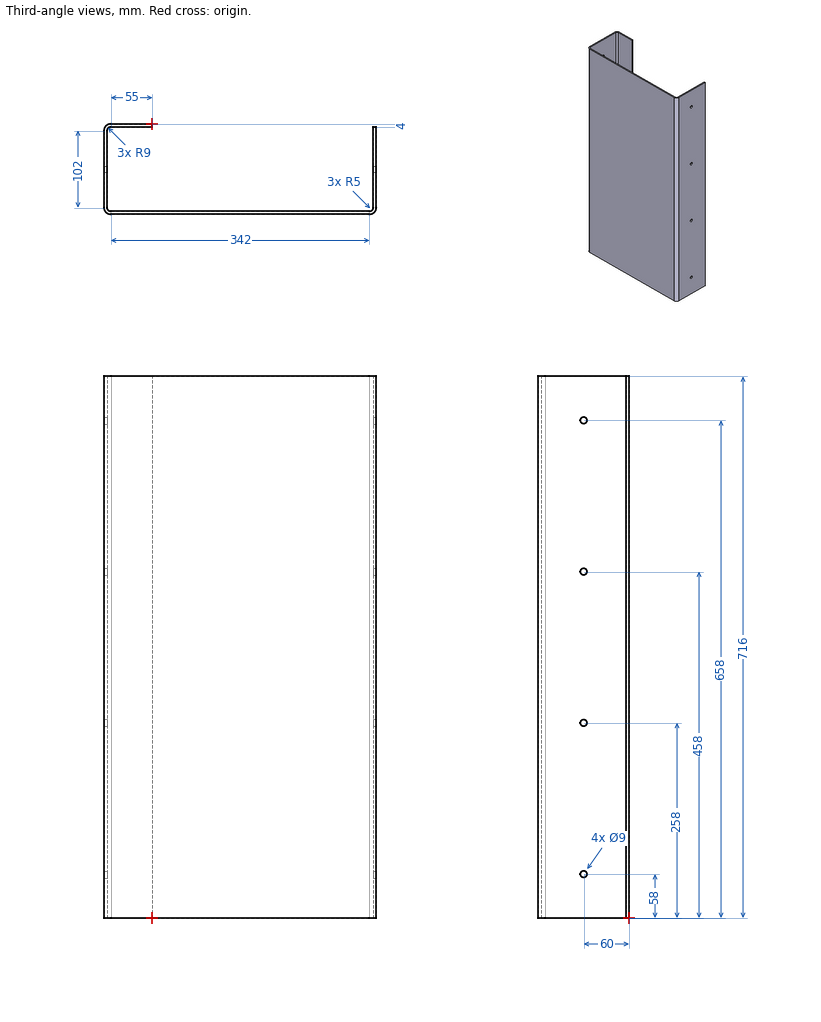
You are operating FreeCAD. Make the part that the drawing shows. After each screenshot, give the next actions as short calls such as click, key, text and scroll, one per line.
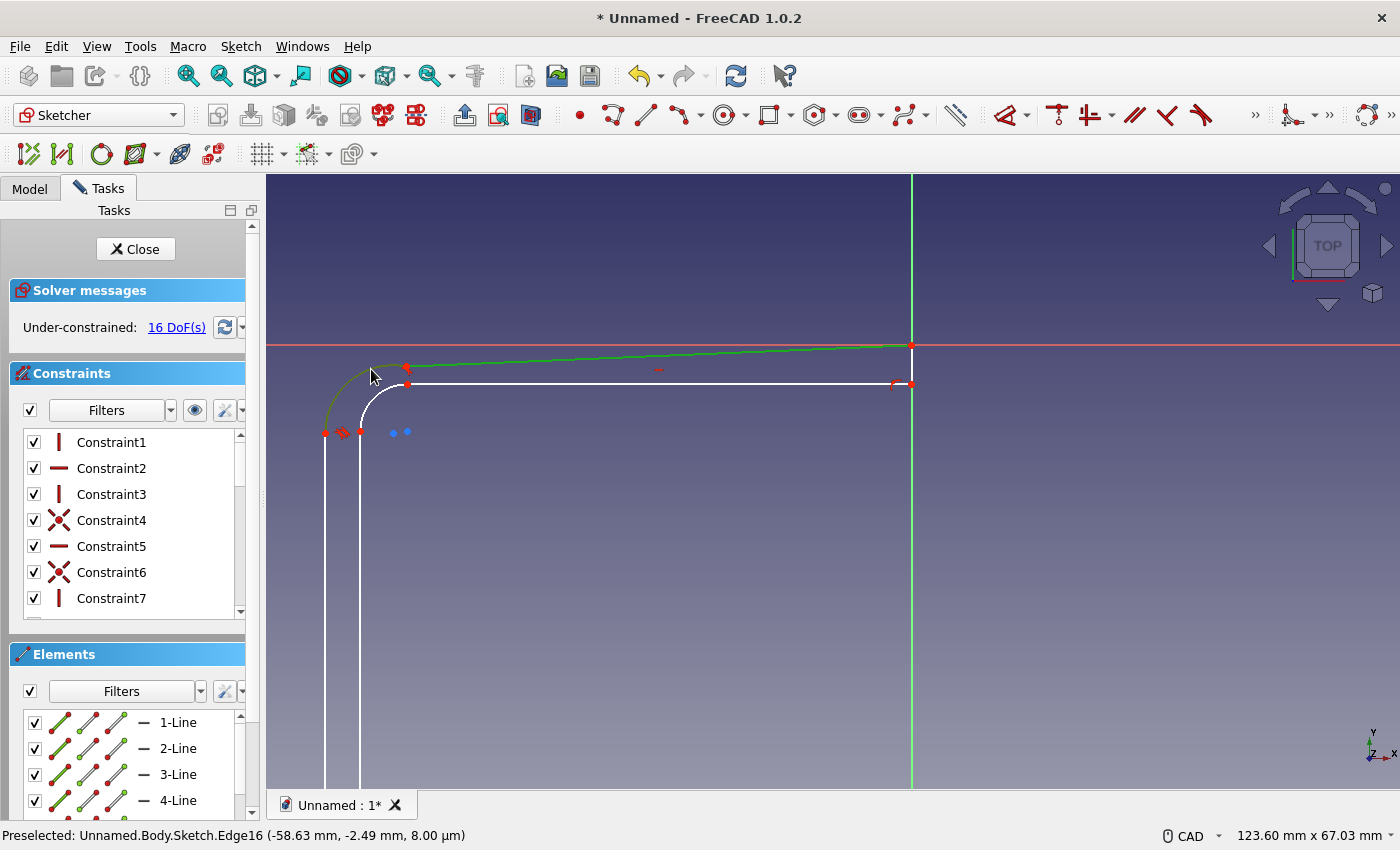
click(1201, 116)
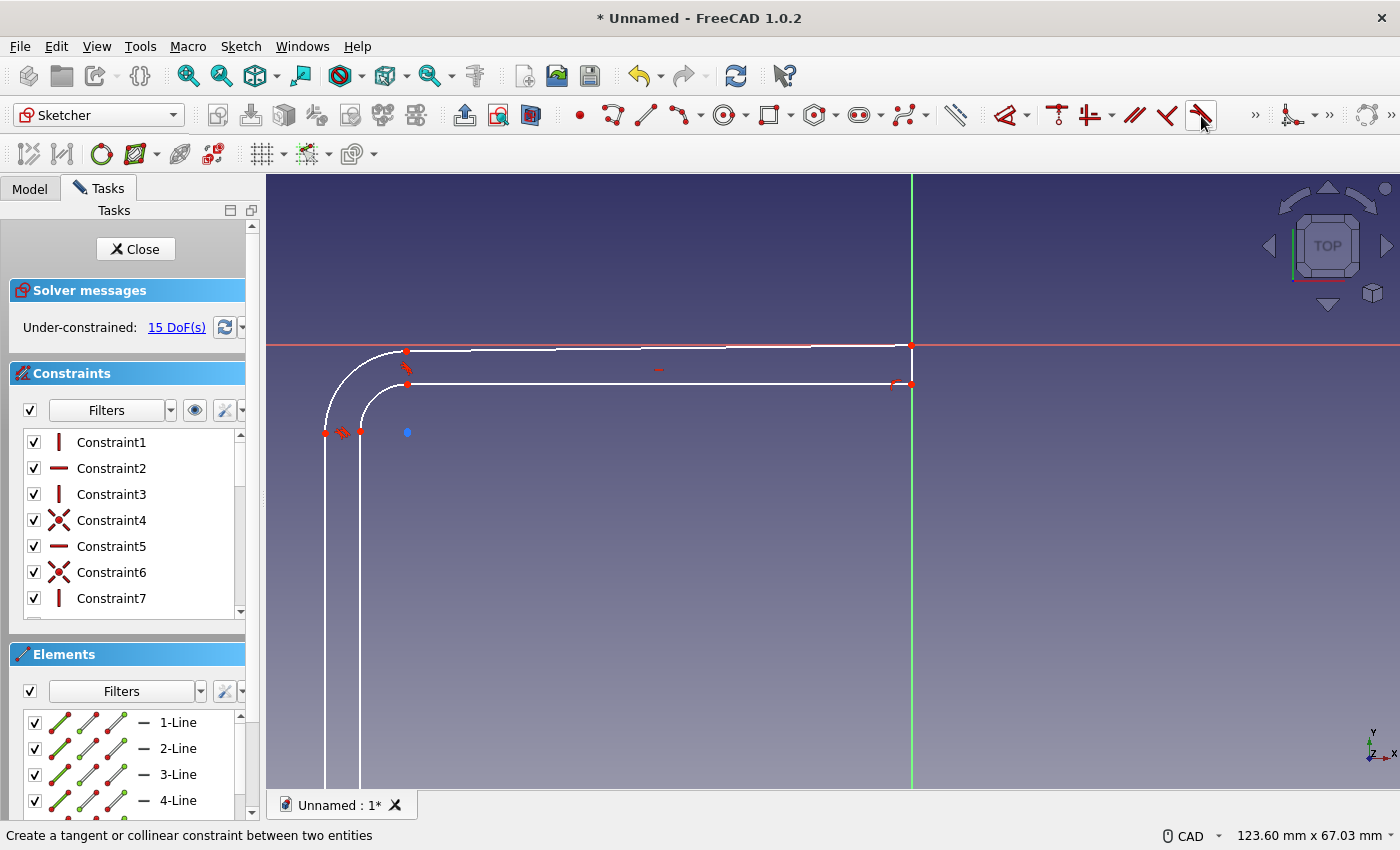
click(760, 347)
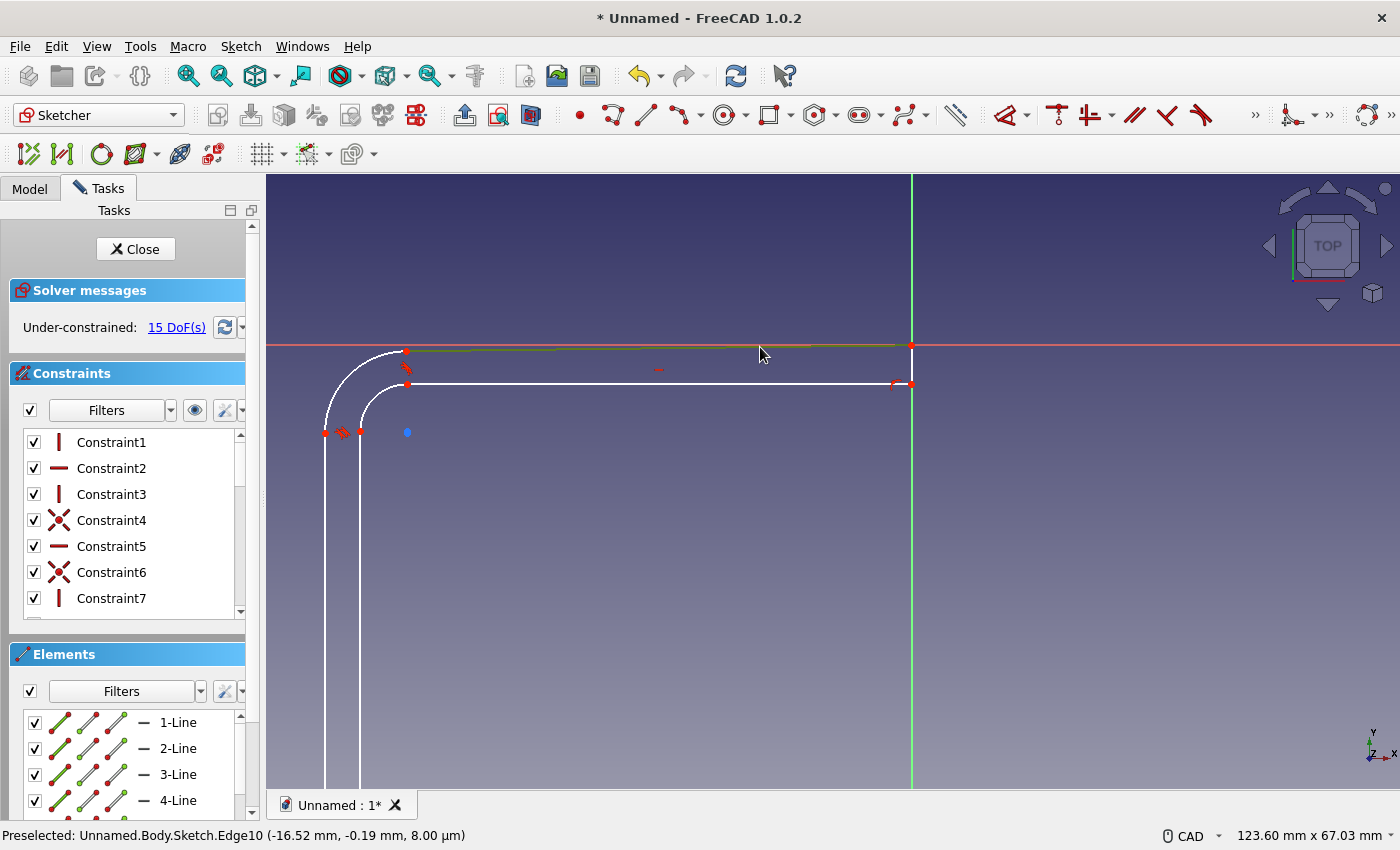
key(h)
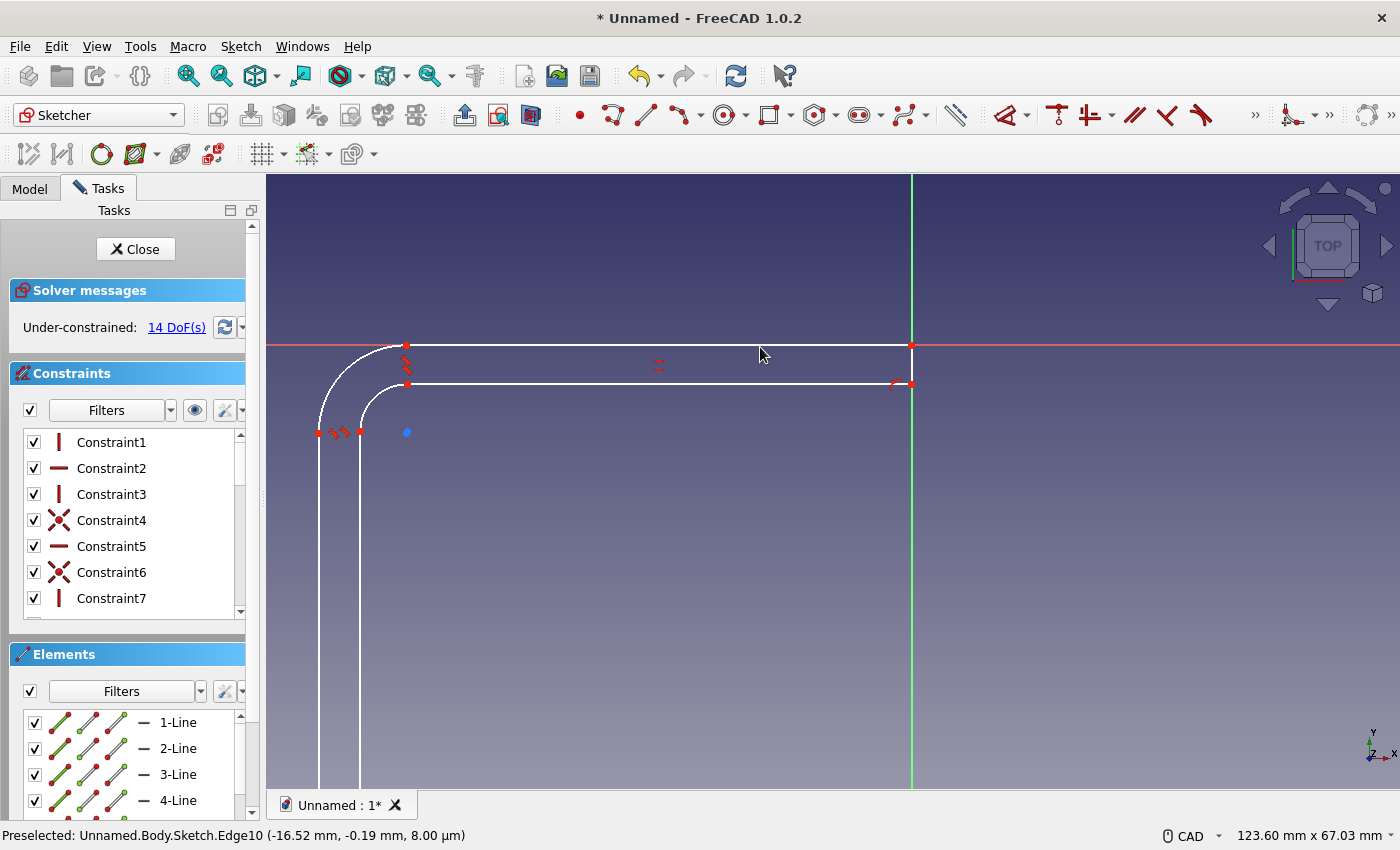
scroll(458, 377, down, 8)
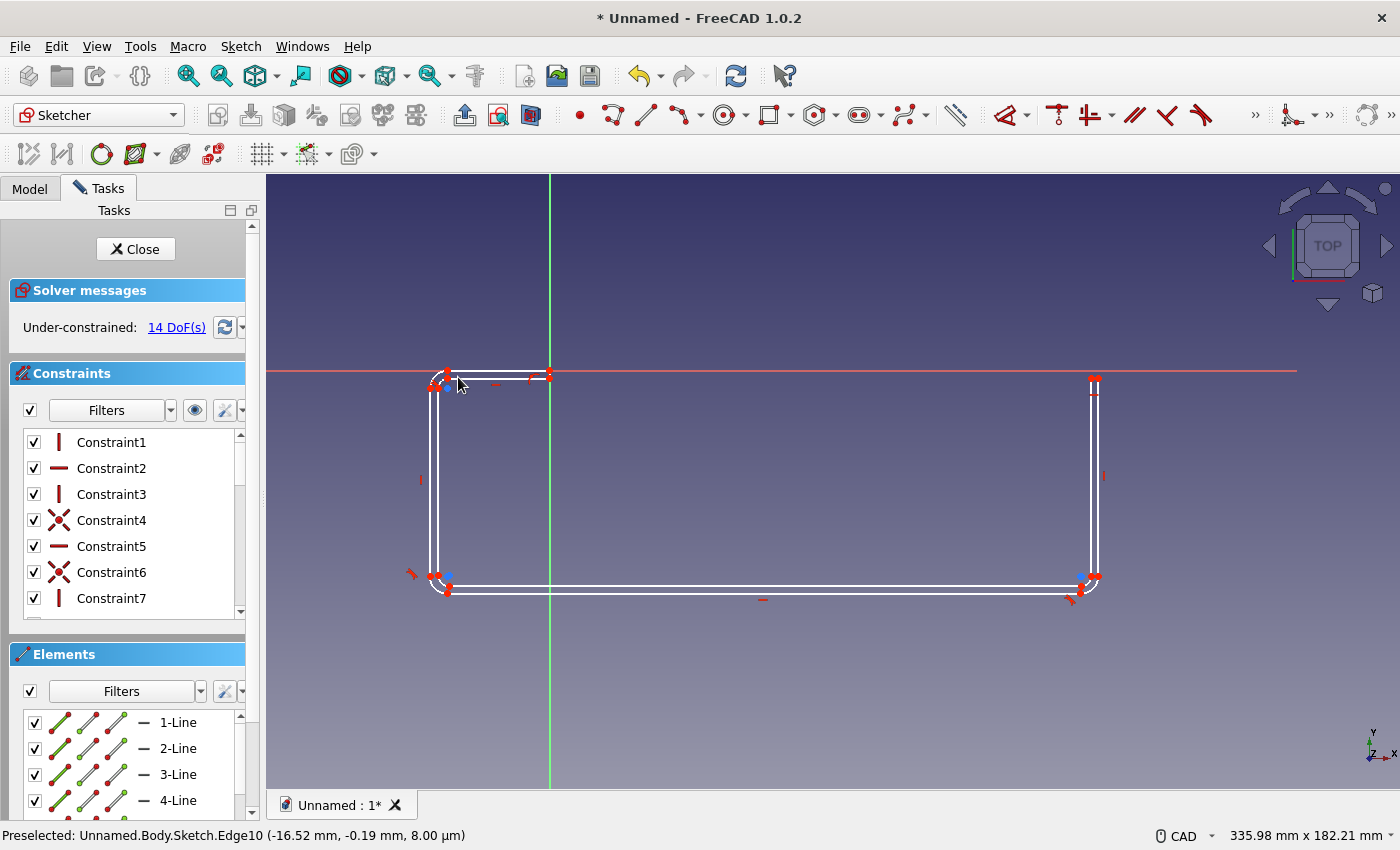
scroll(1089, 592, up, 4)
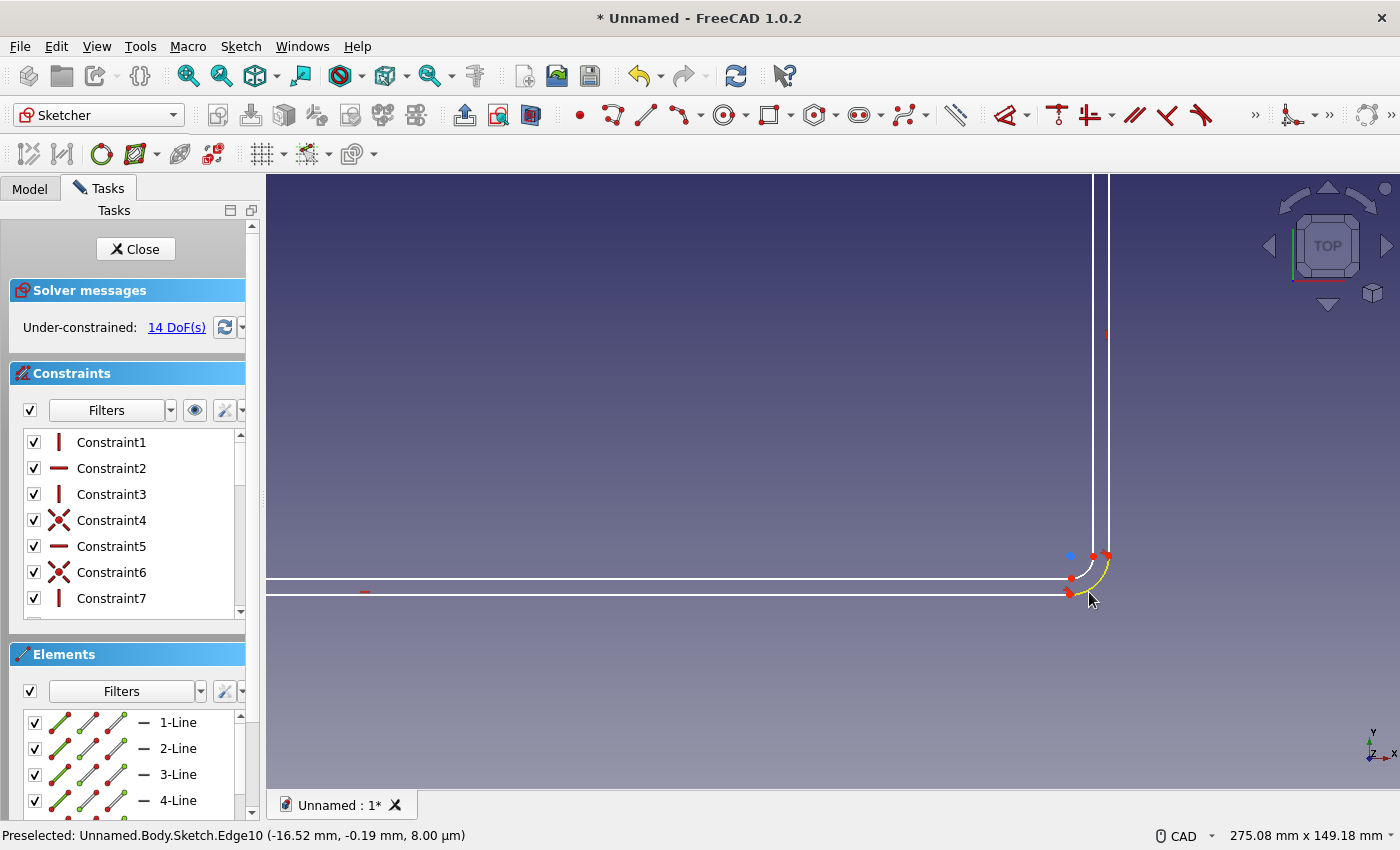
click(1087, 591)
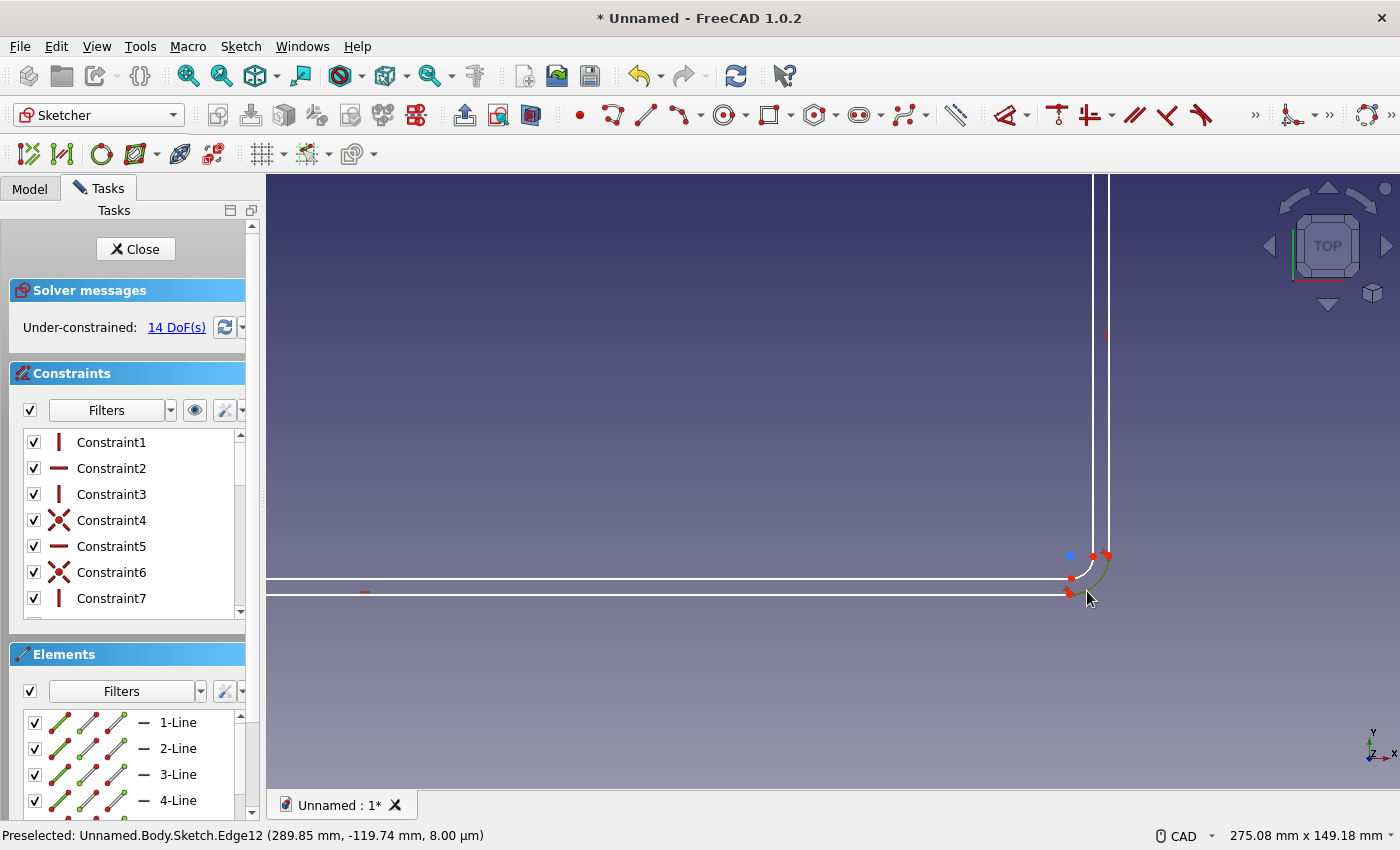
scroll(1081, 576, up, 2)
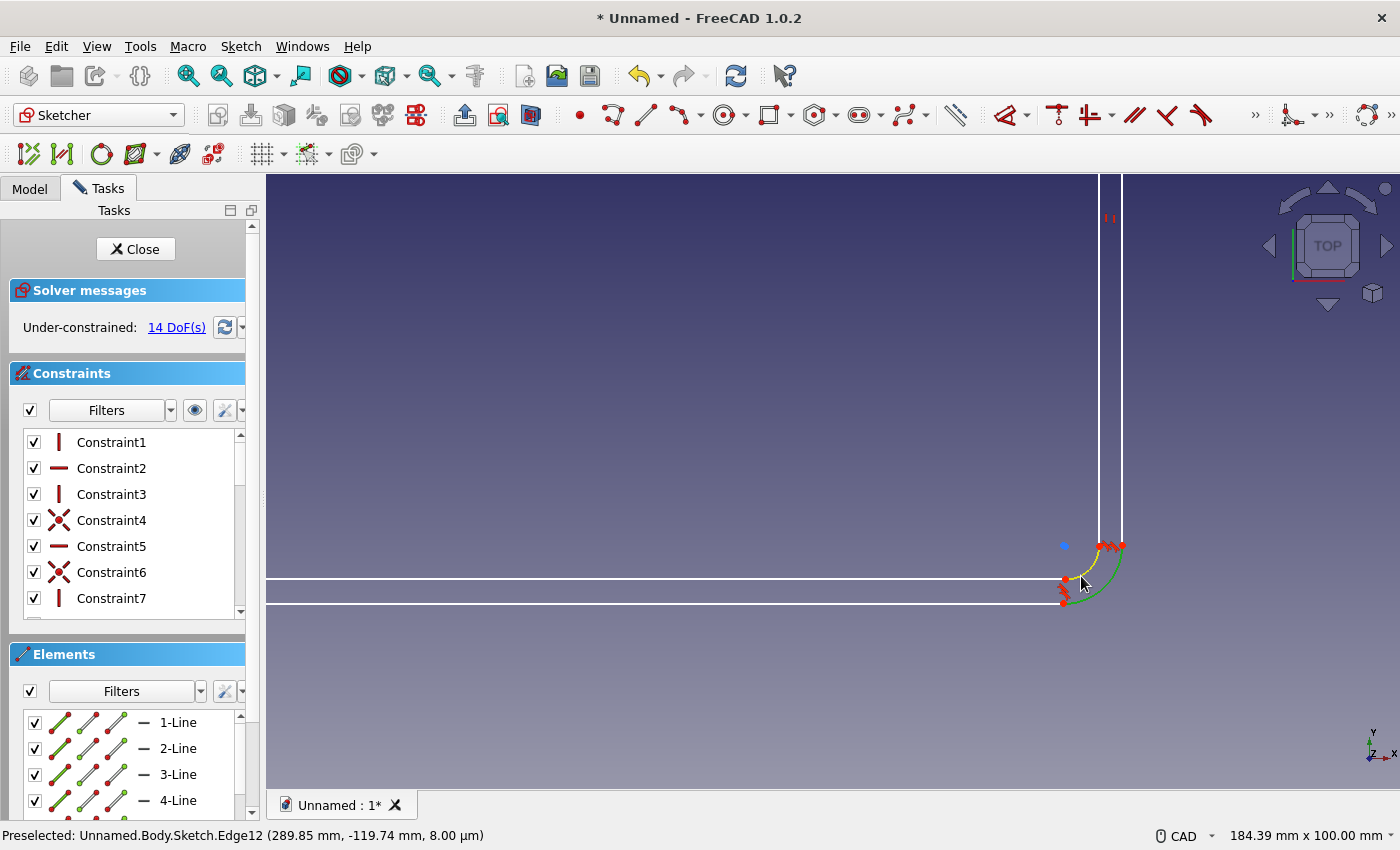
click(1081, 576)